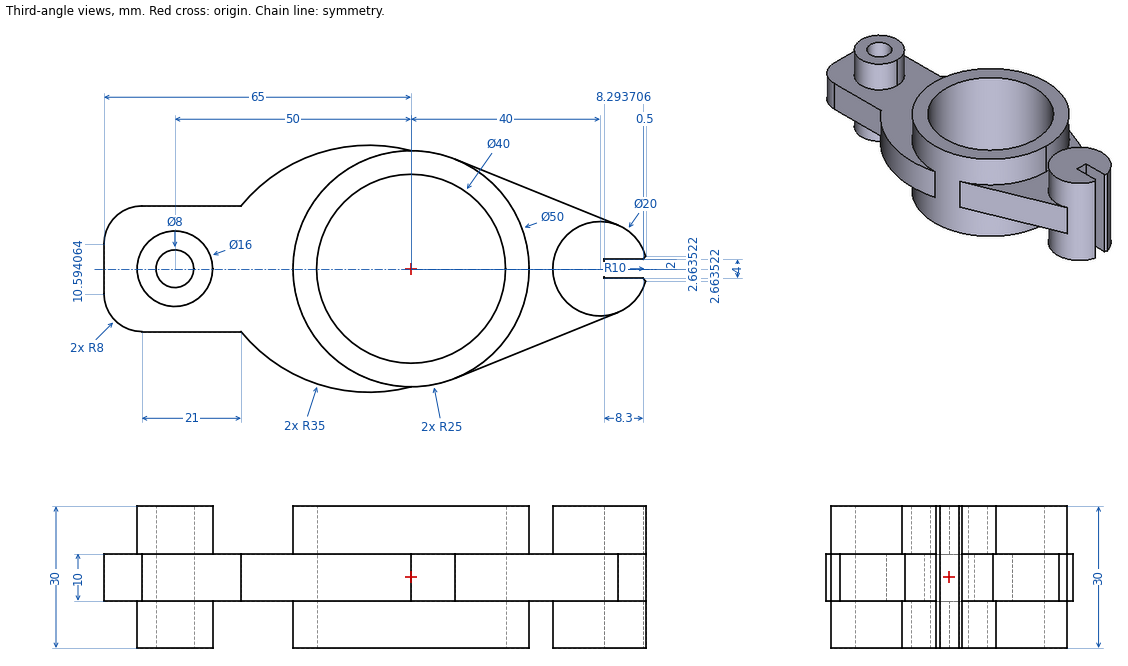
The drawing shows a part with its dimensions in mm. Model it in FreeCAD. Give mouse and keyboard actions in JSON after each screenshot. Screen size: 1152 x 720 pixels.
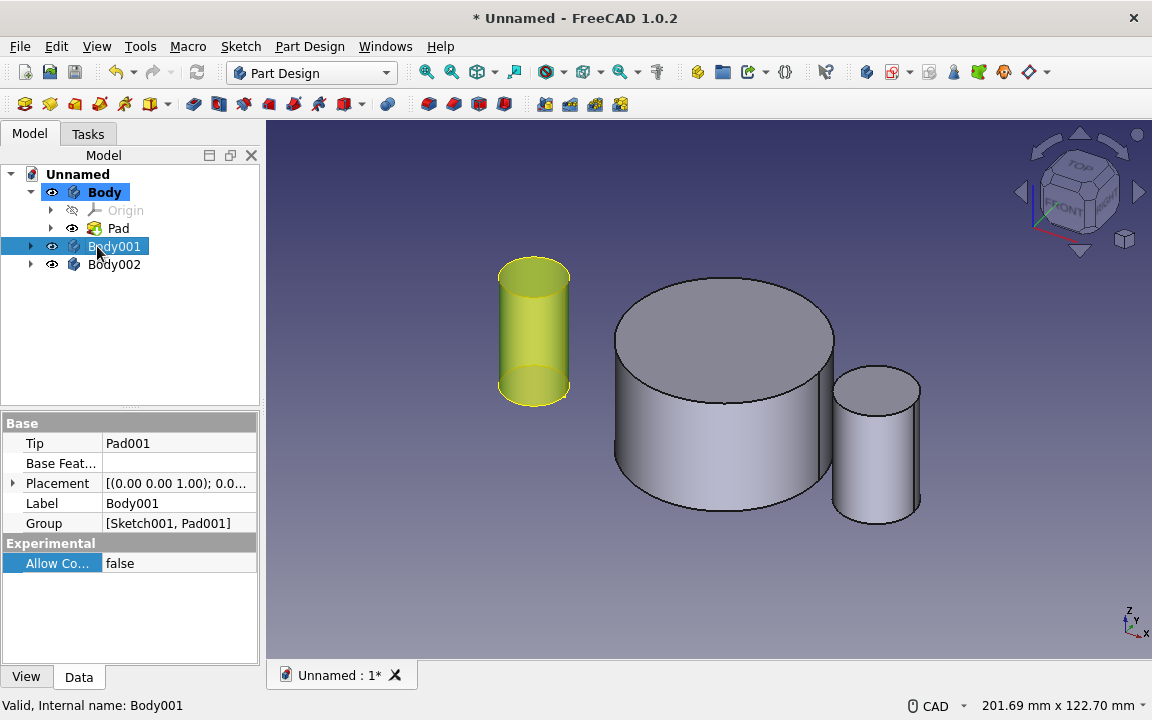
{"action": "left_click", "coordinate": [388, 104]}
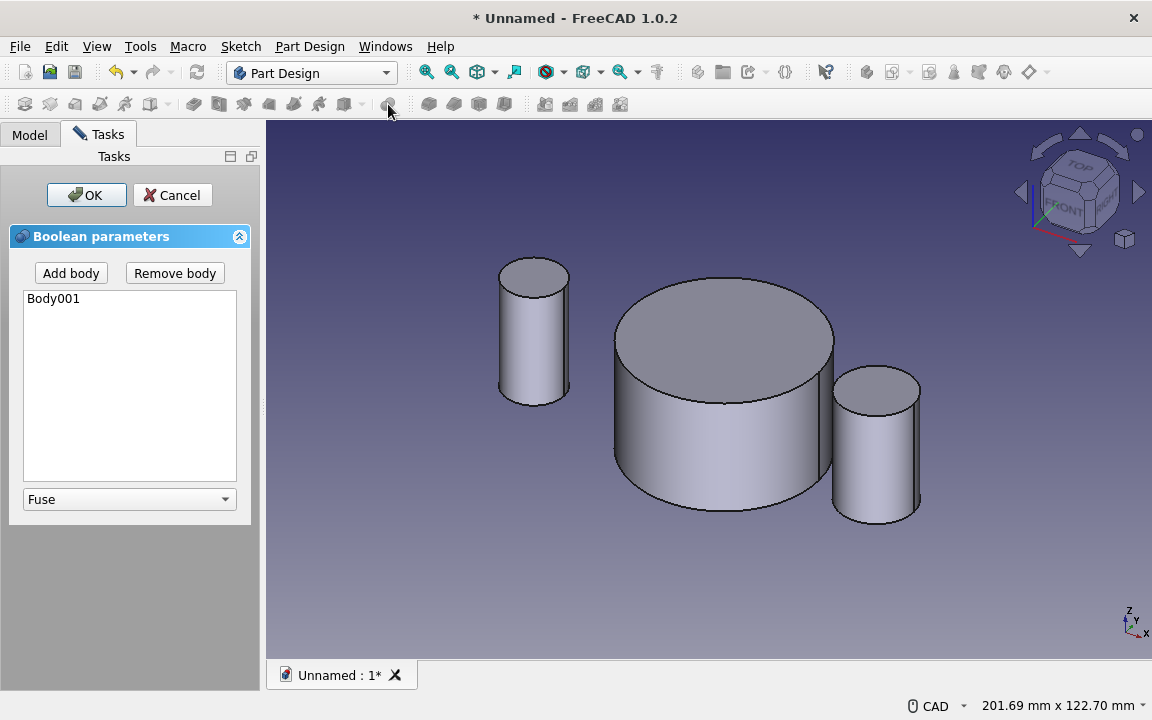
{"action": "left_click", "coordinate": [87, 195]}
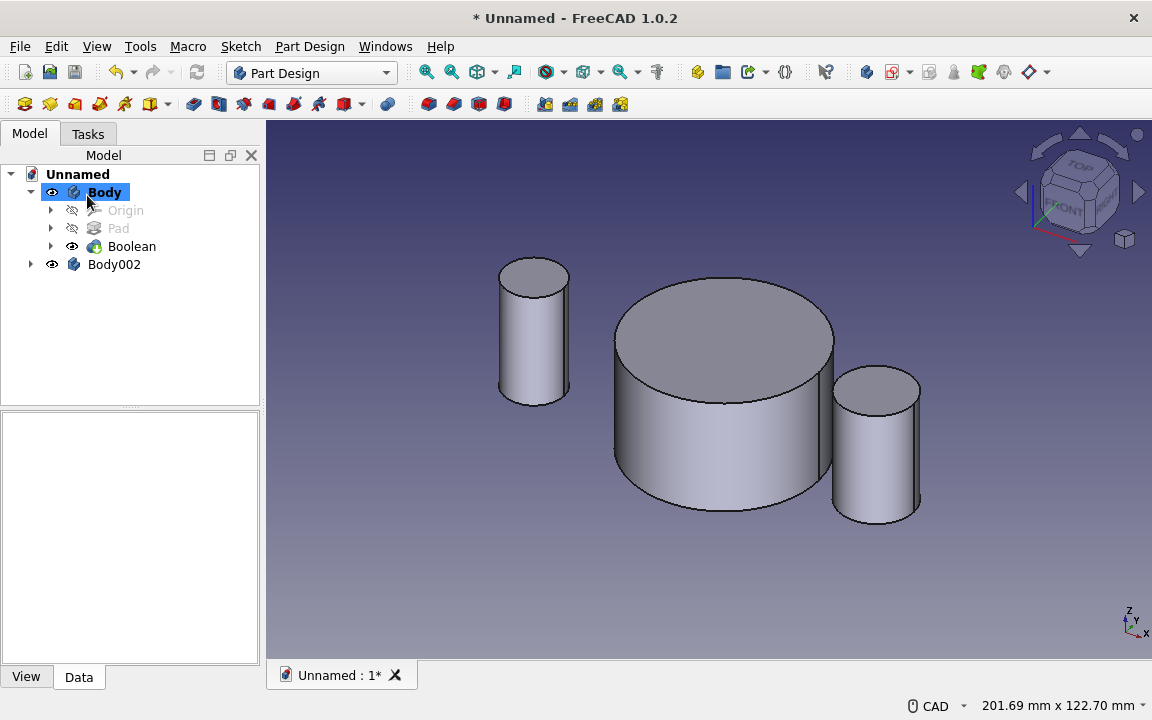
{"action": "left_click", "coordinate": [97, 264]}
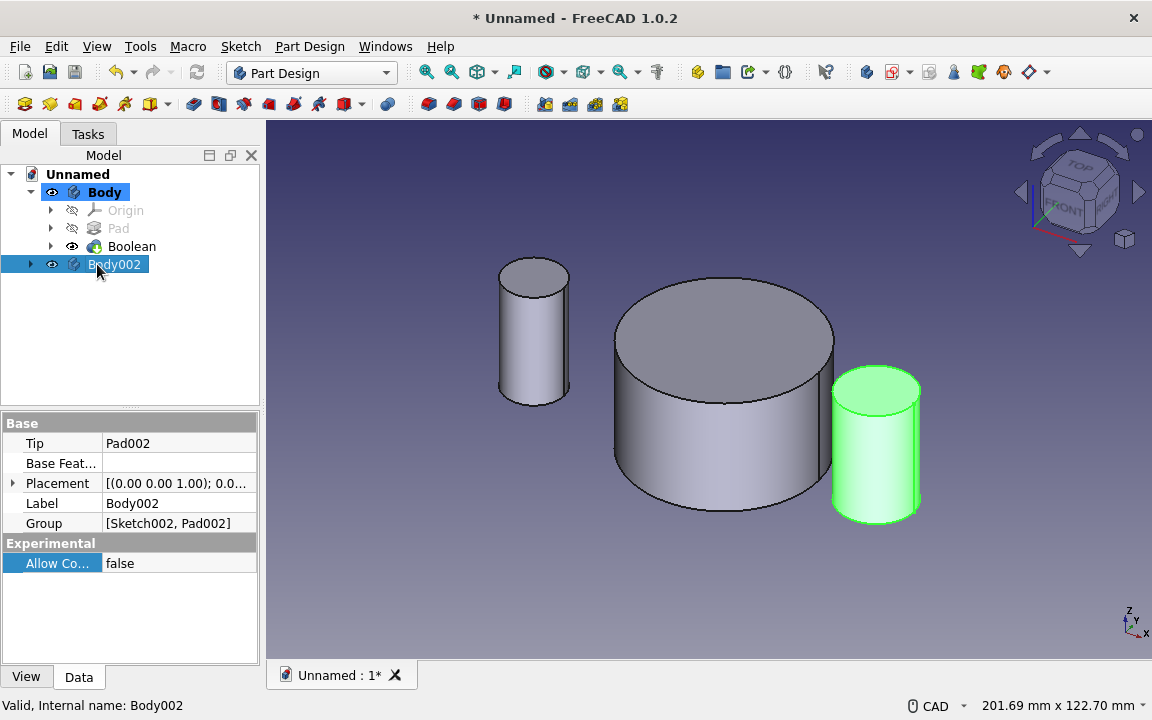
{"action": "left_click", "coordinate": [388, 104]}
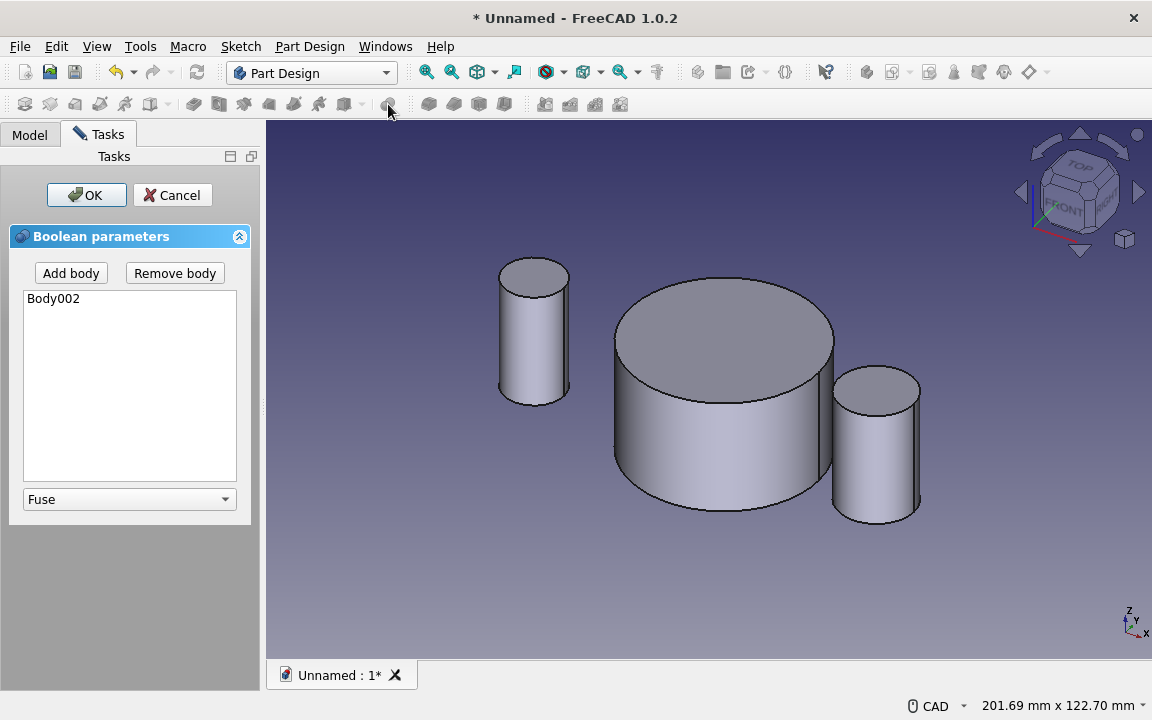
{"action": "left_click", "coordinate": [87, 195]}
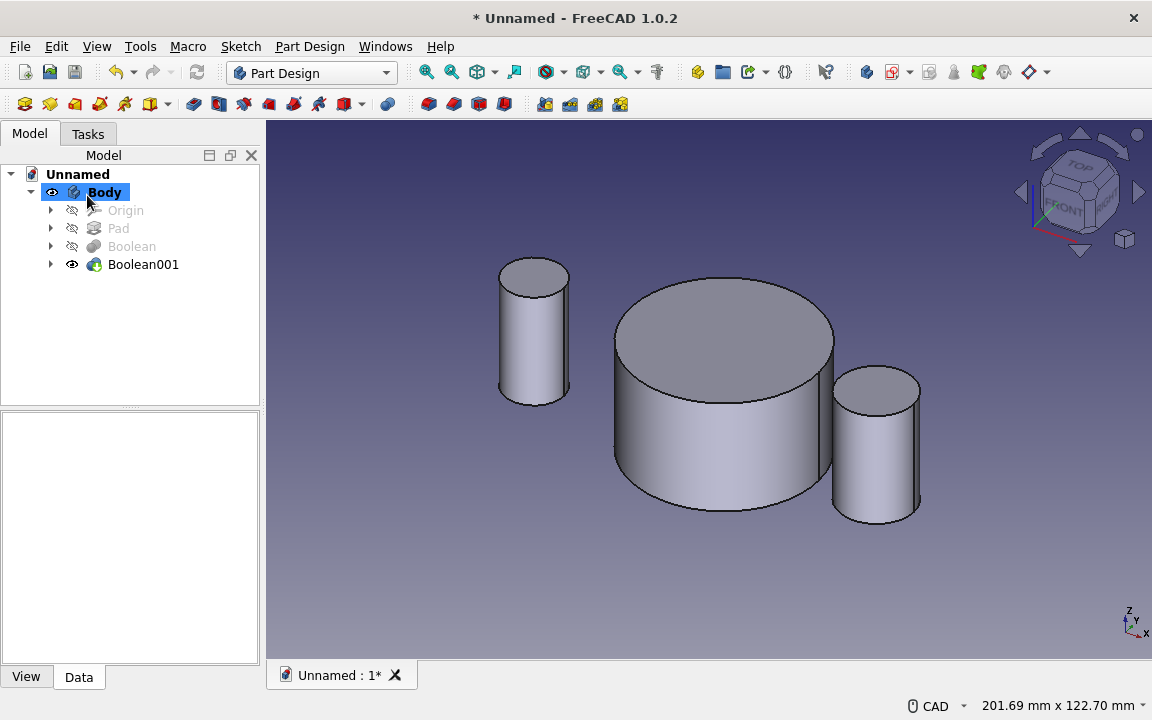
{"action": "left_click", "coordinate": [892, 72]}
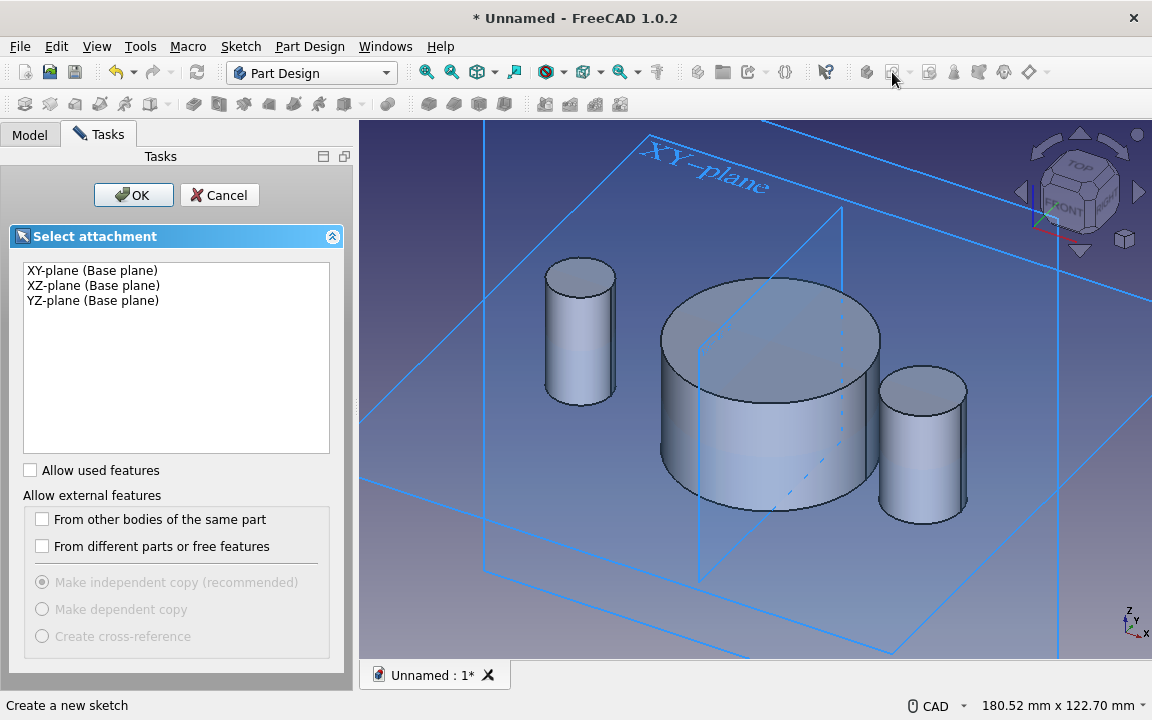
{"action": "left_click", "coordinate": [84, 270]}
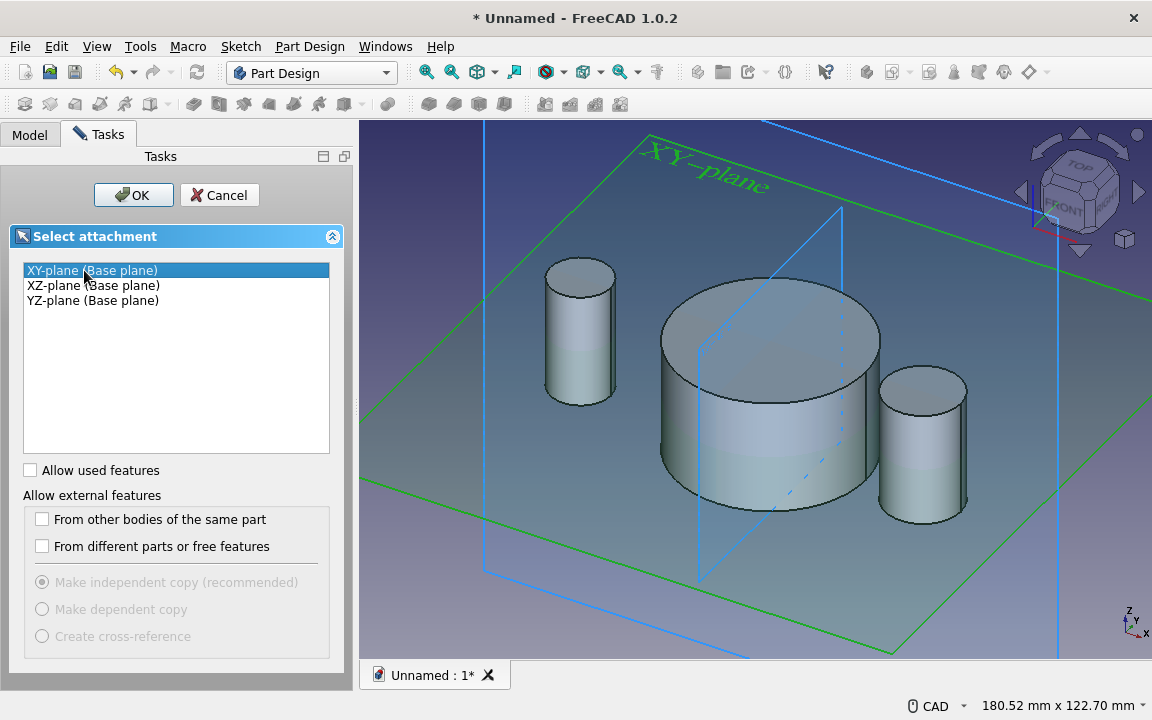
{"action": "left_click", "coordinate": [134, 195]}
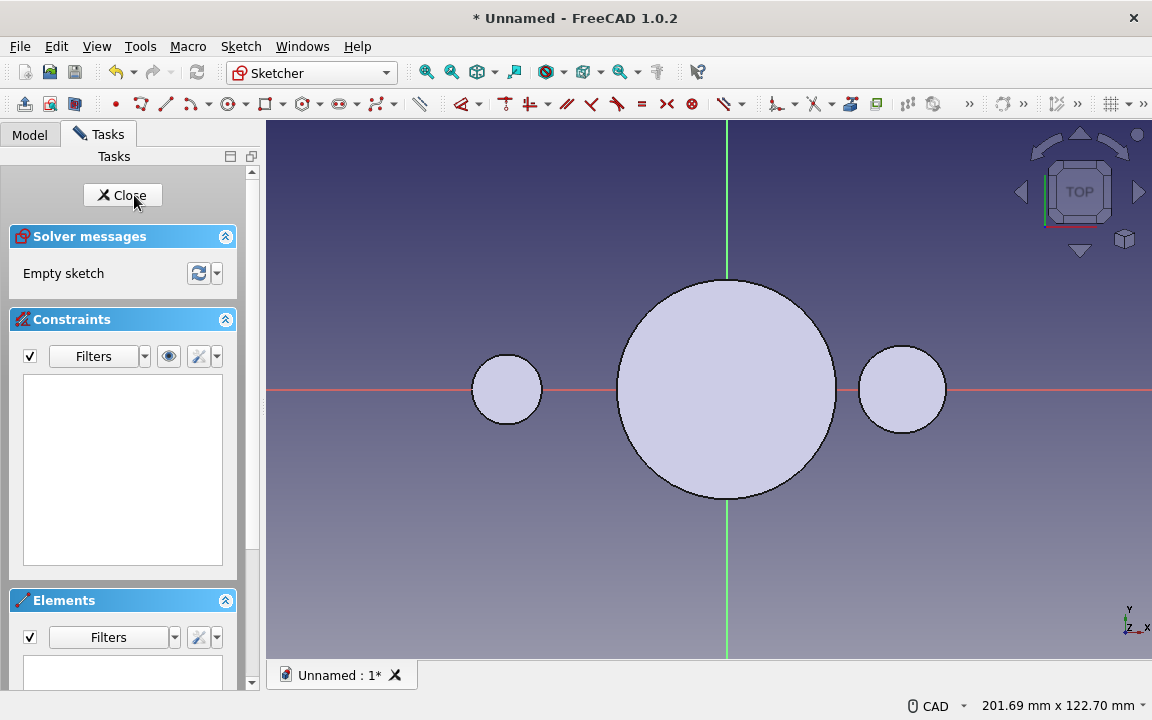
{"action": "key", "text": "q s"}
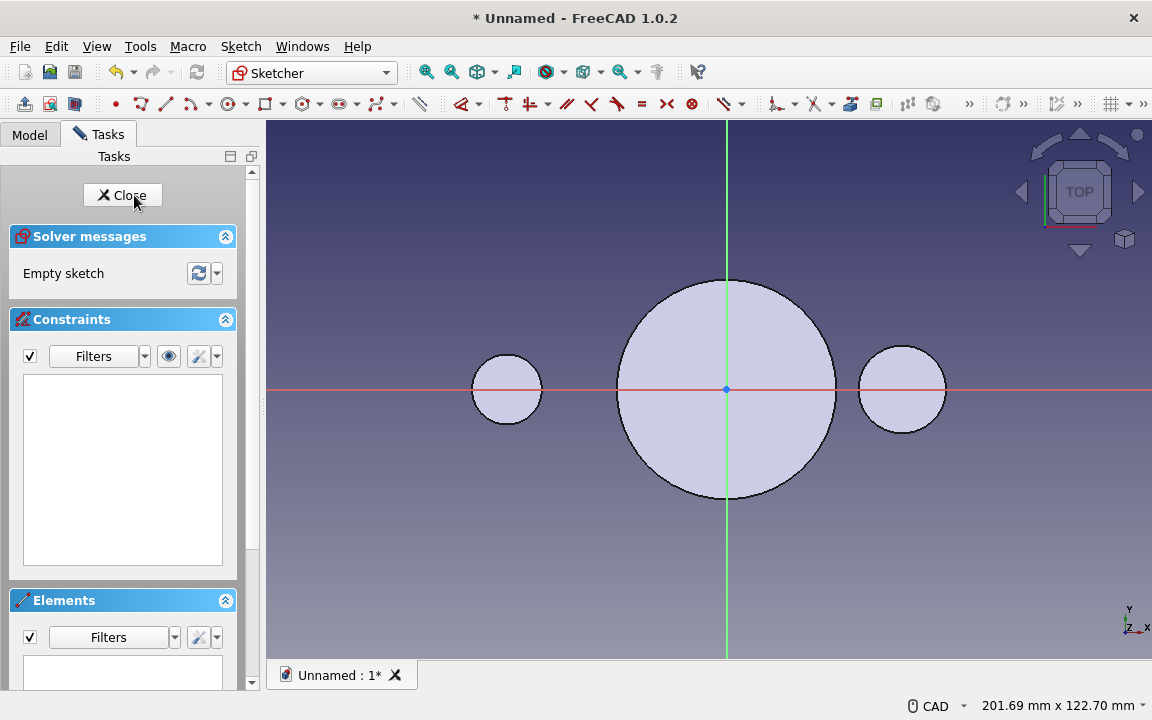
{"action": "left_click", "coordinate": [166, 104]}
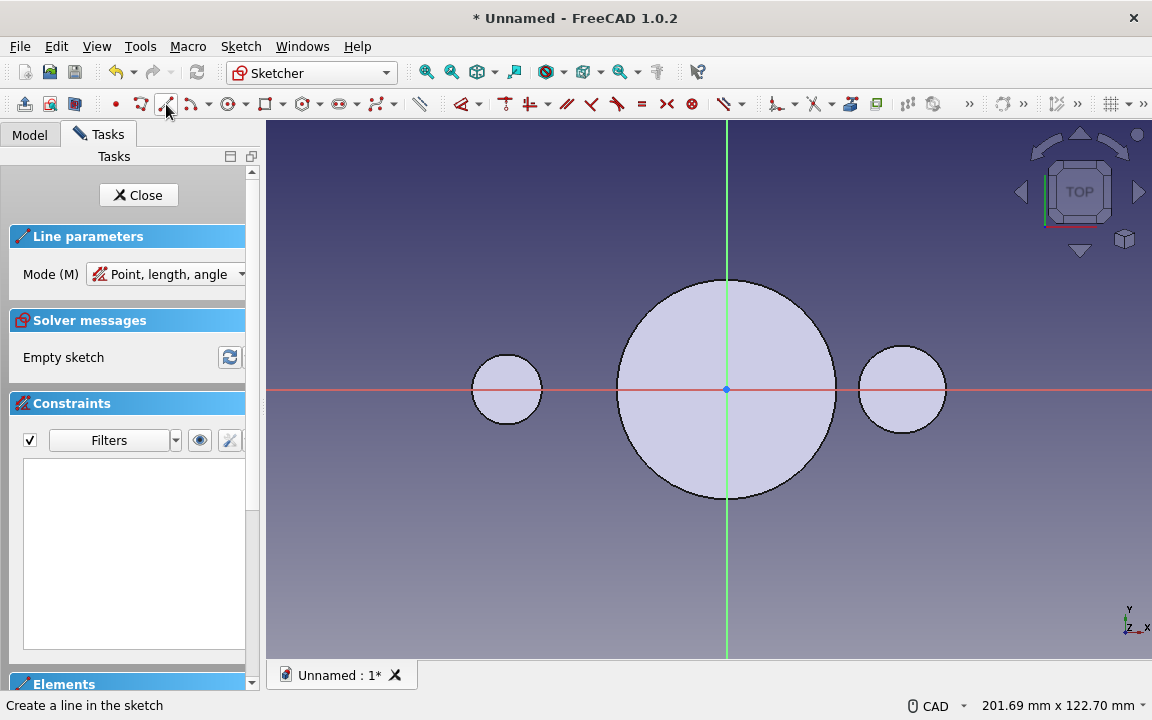
{"action": "left_click", "coordinate": [441, 366]}
{"action": "left_click", "coordinate": [441, 413]}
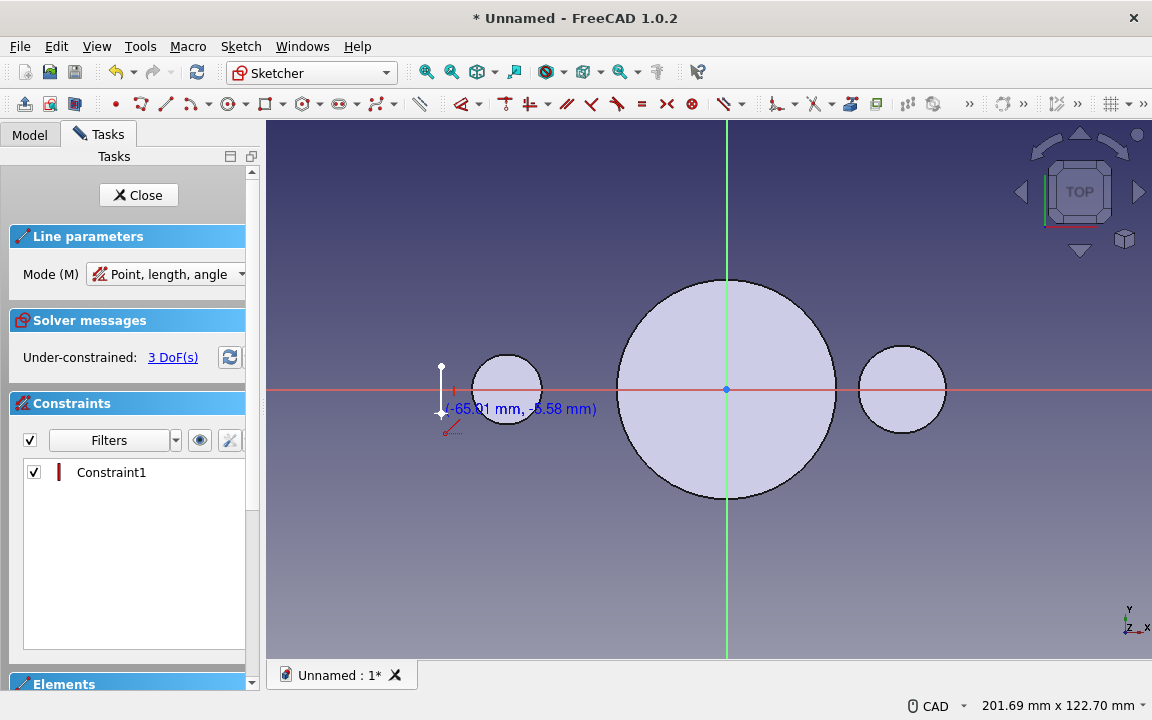
{"action": "left_click", "coordinate": [476, 448]}
{"action": "left_click", "coordinate": [568, 448]}